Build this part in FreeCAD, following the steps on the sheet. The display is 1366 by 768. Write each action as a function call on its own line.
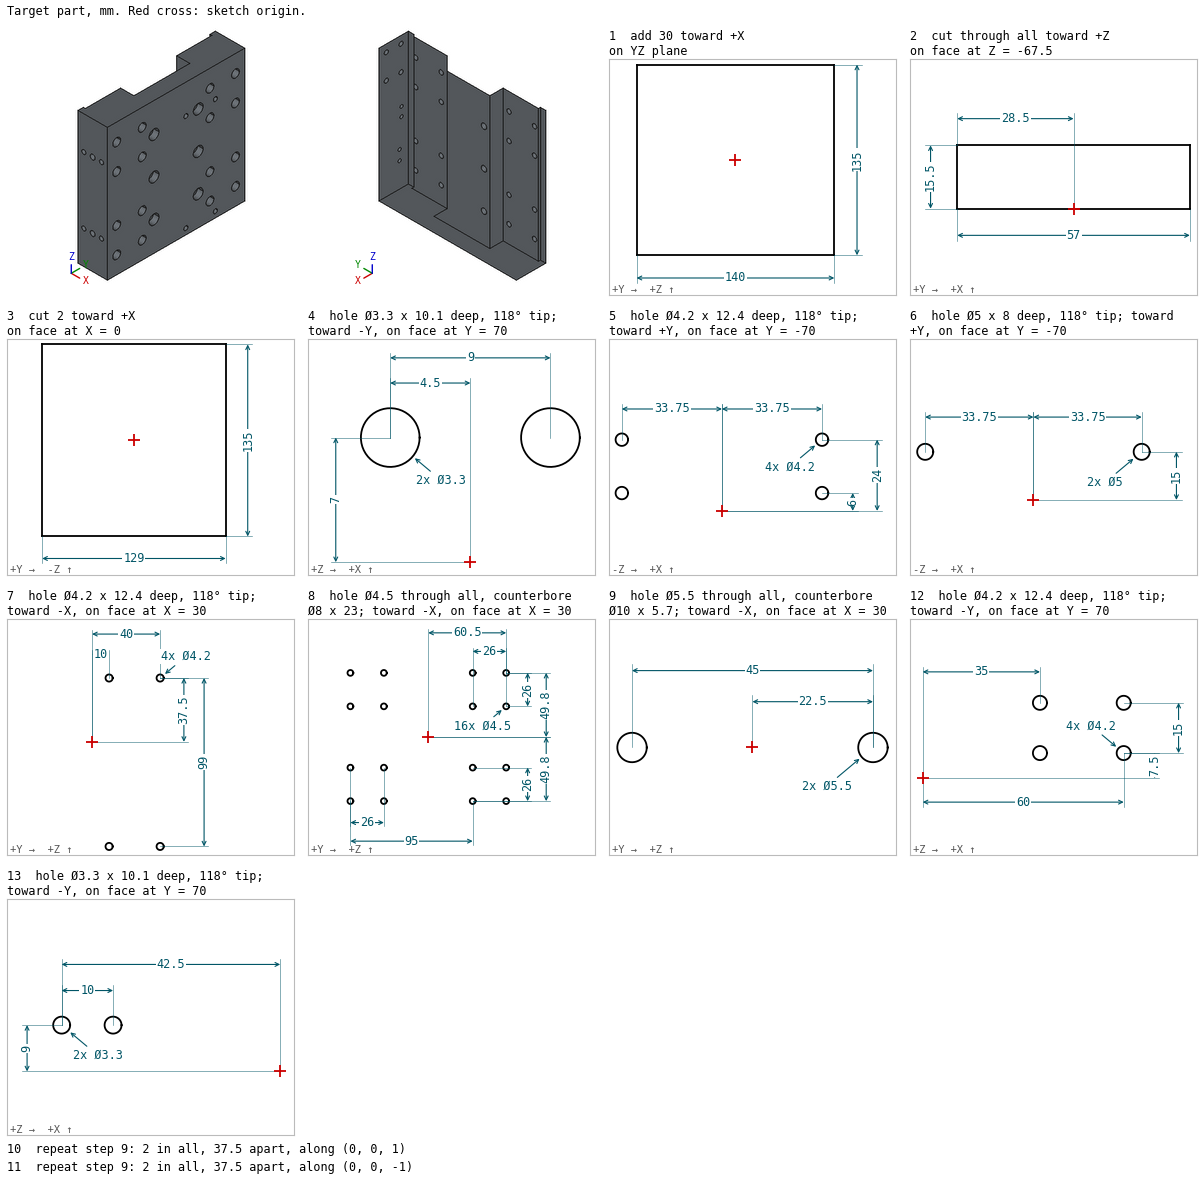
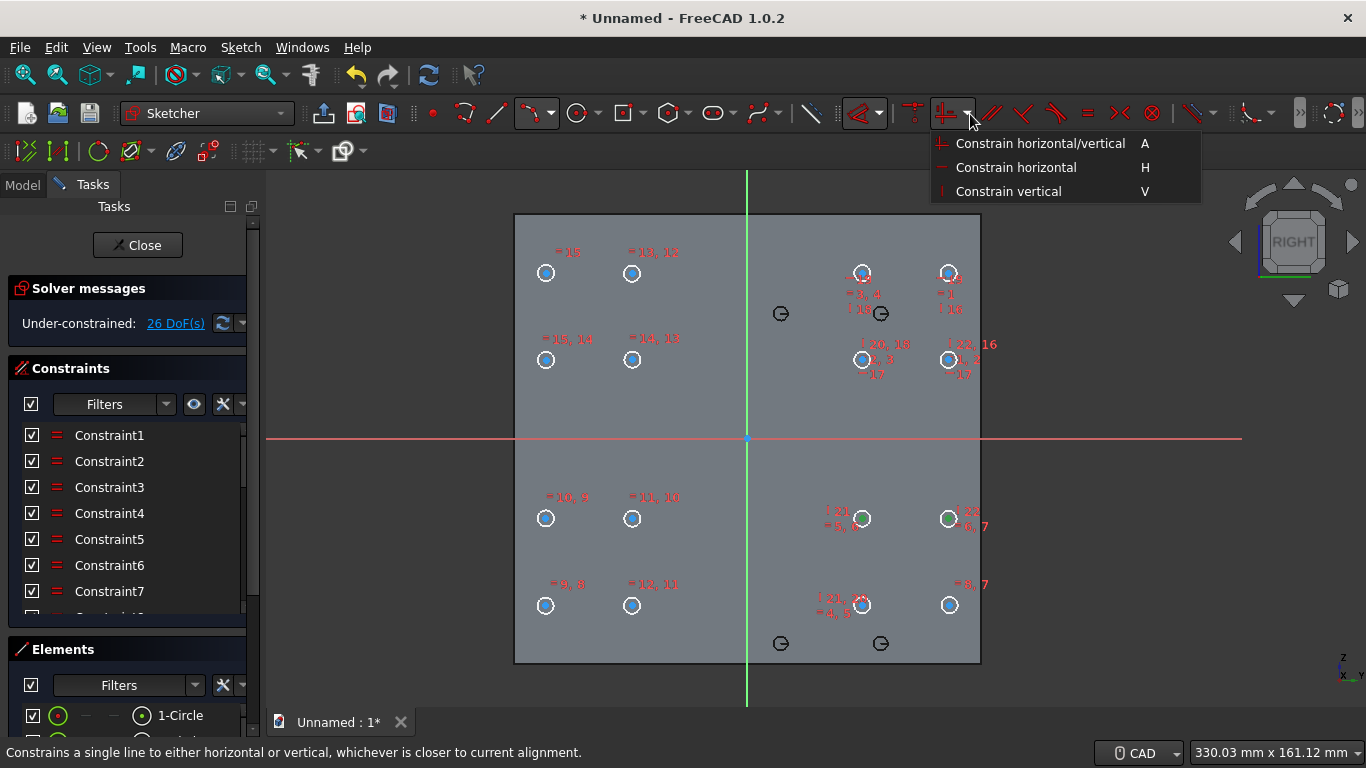
click(1066, 167)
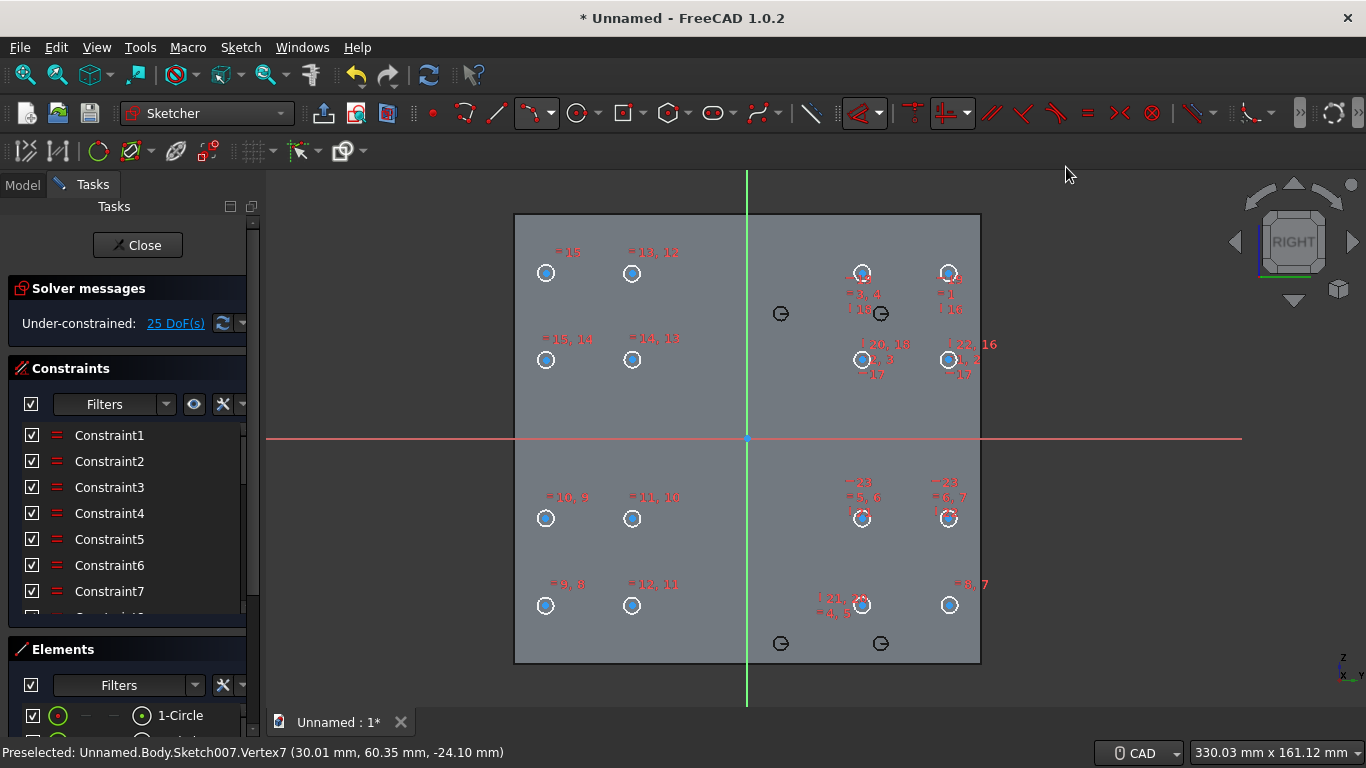
click(949, 519)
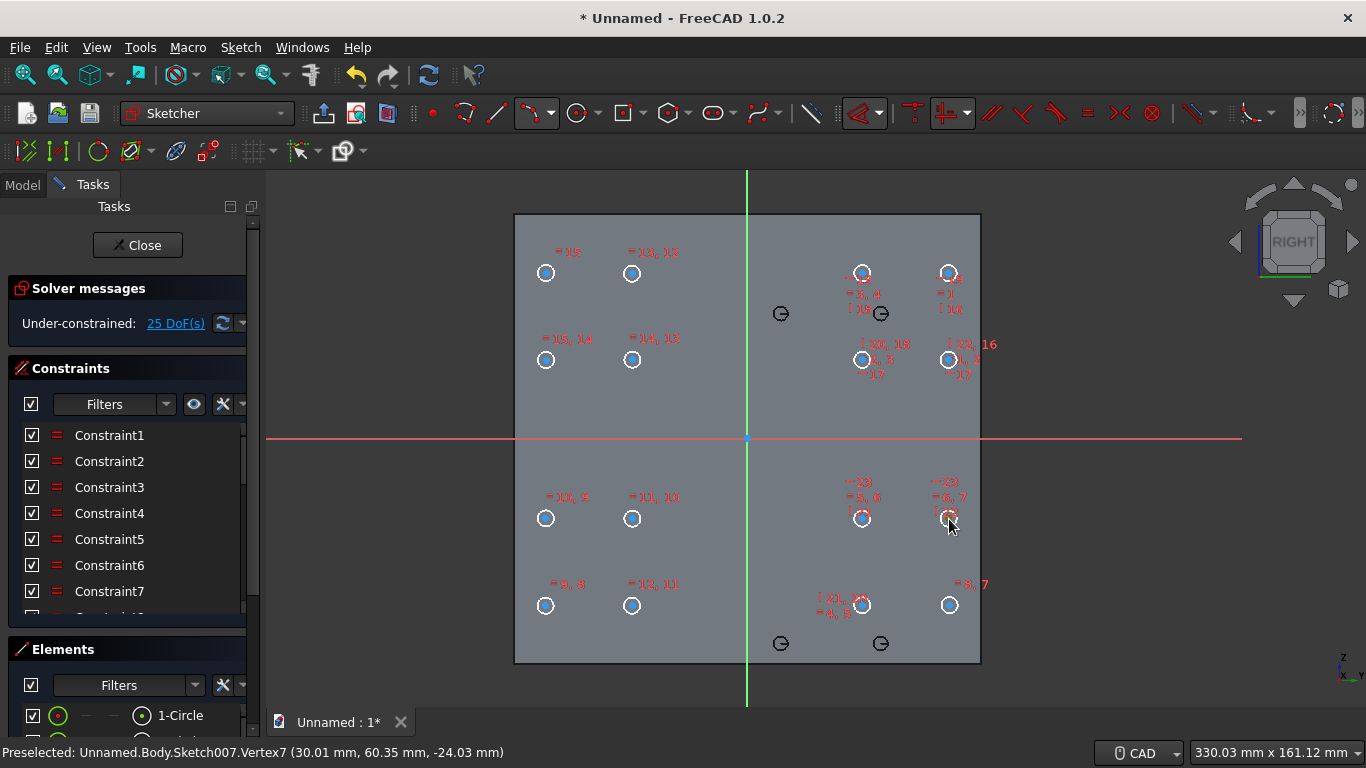
click(950, 605)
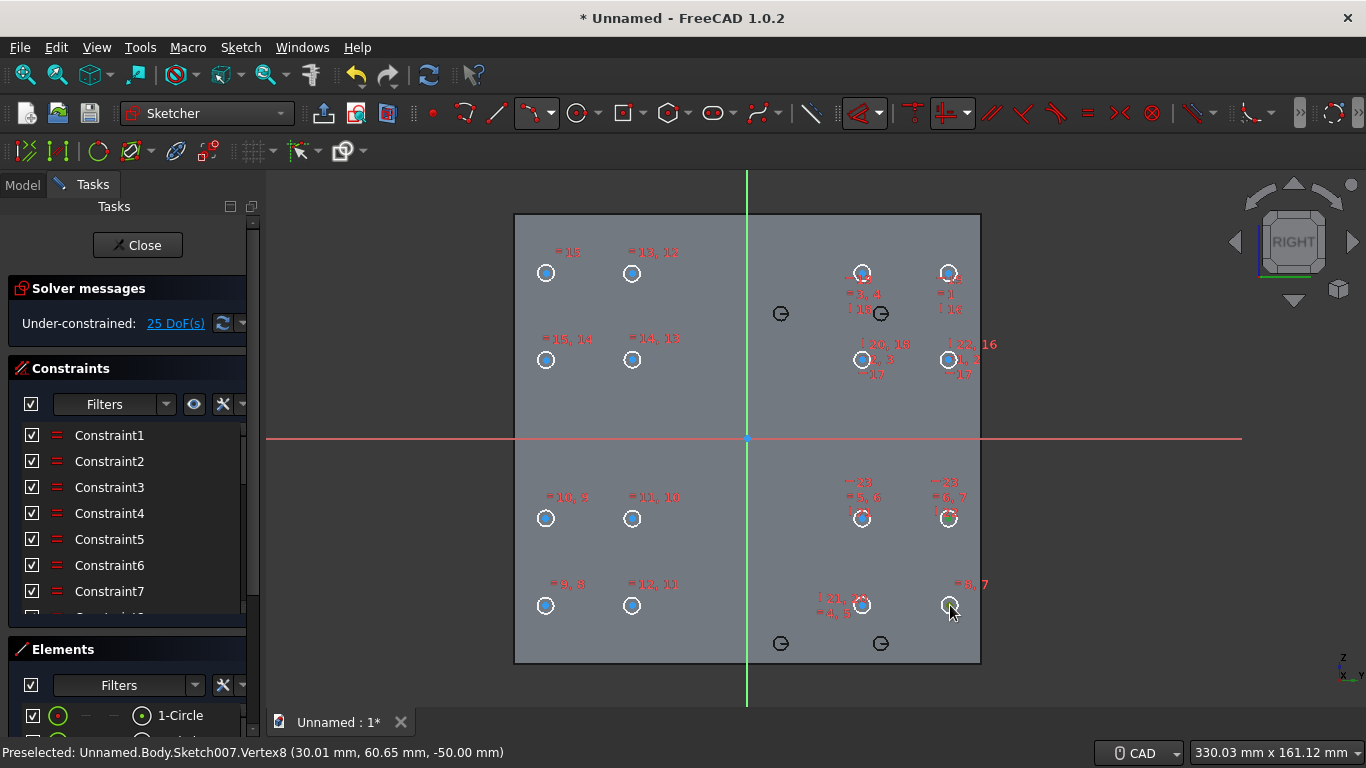
key(v)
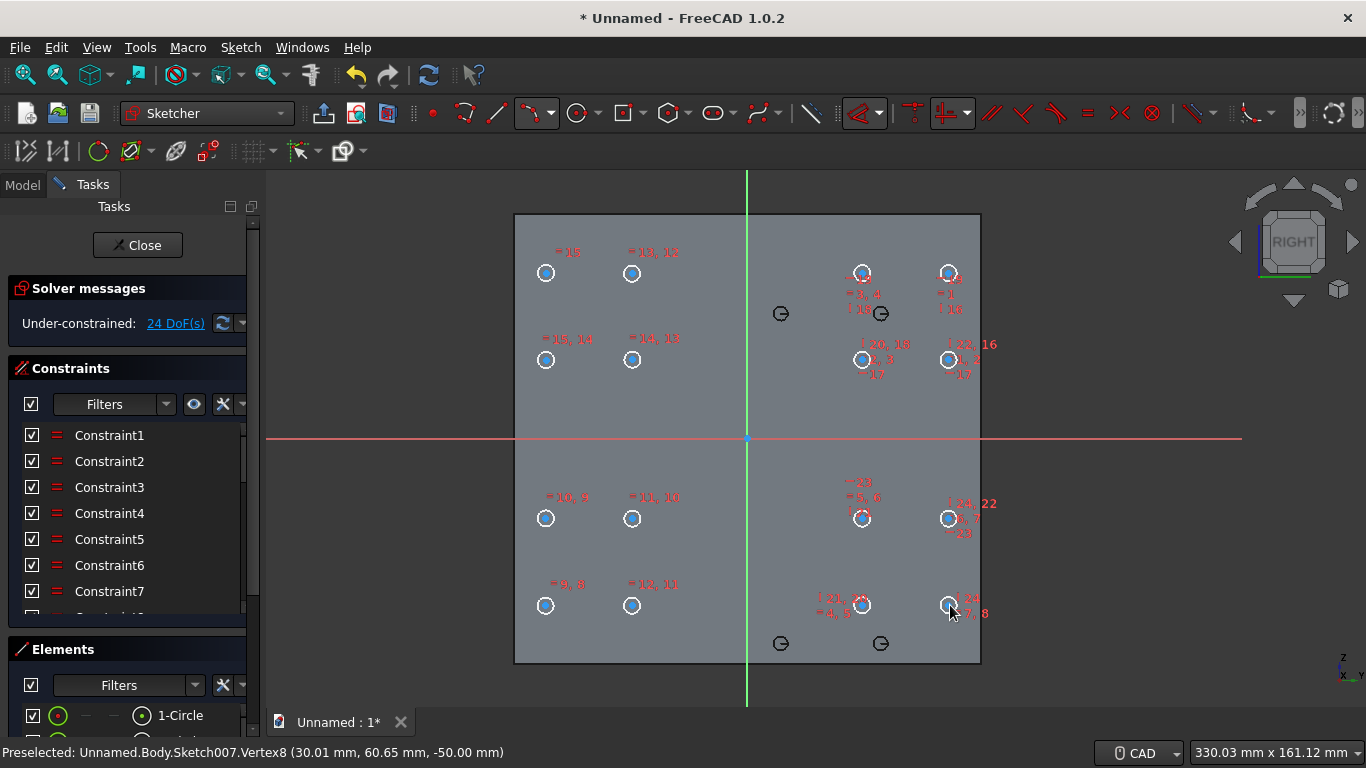
click(862, 605)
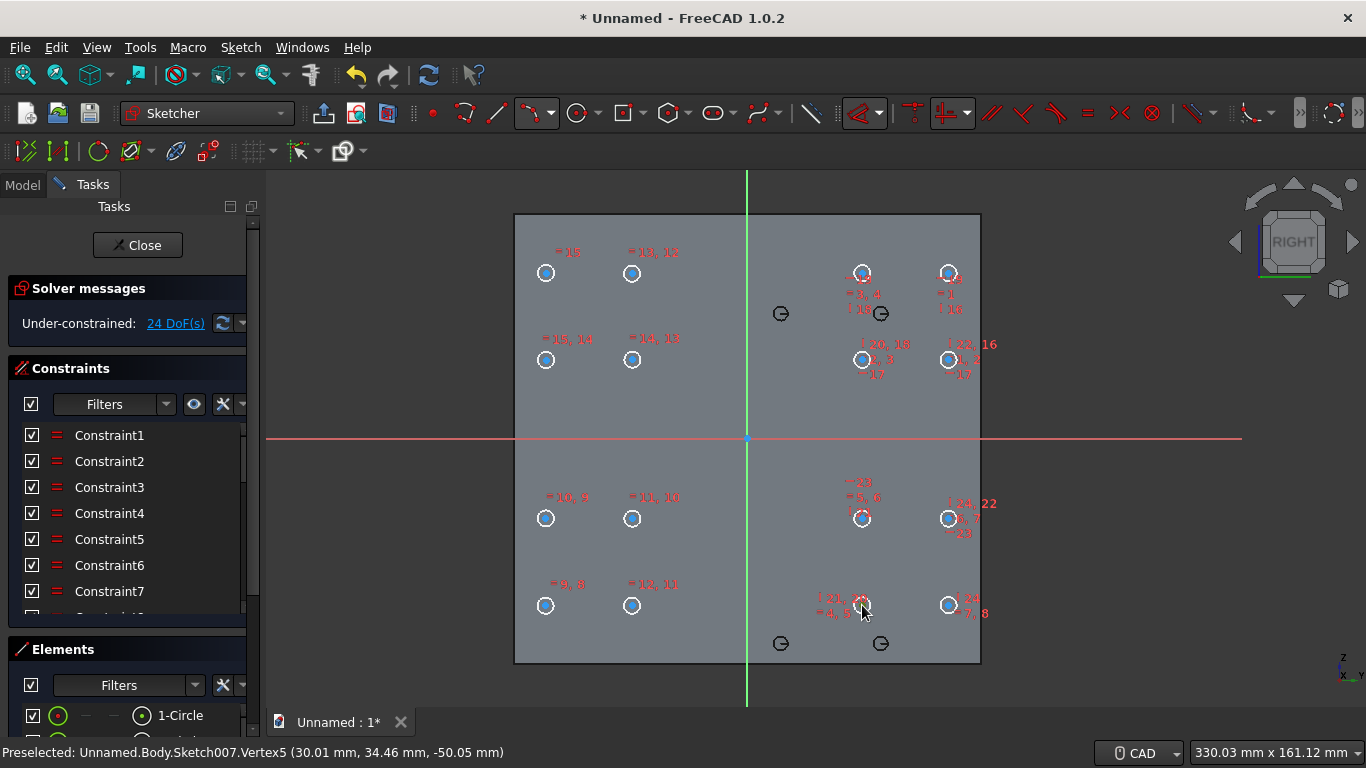
click(949, 605)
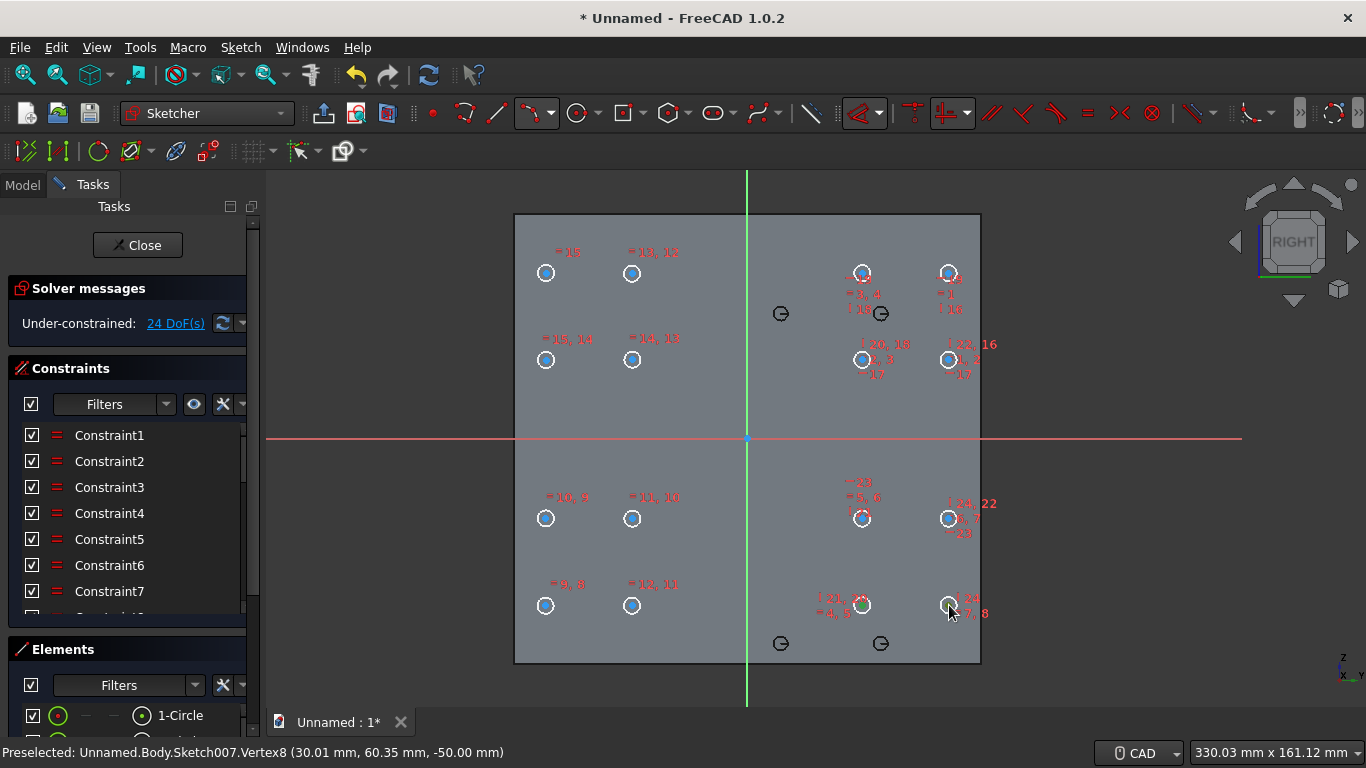
click(970, 114)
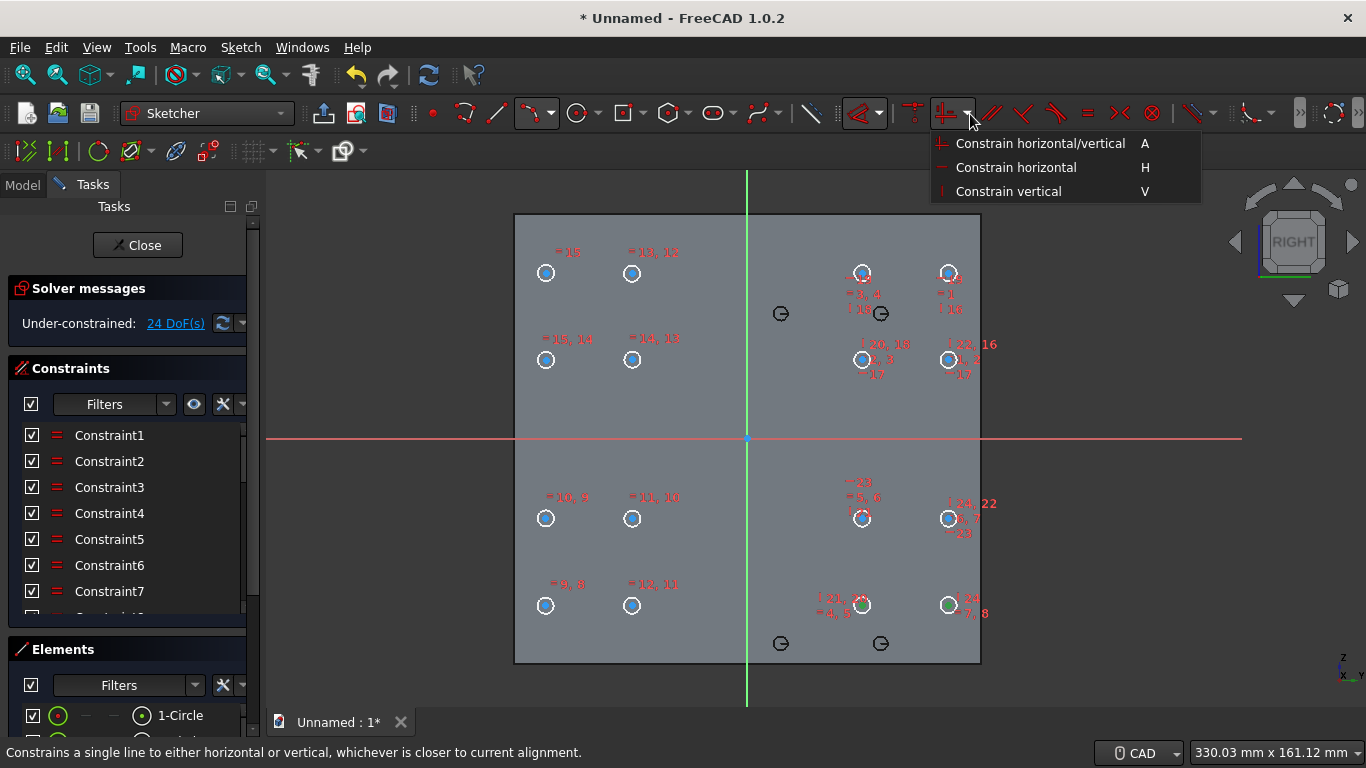
click(1066, 167)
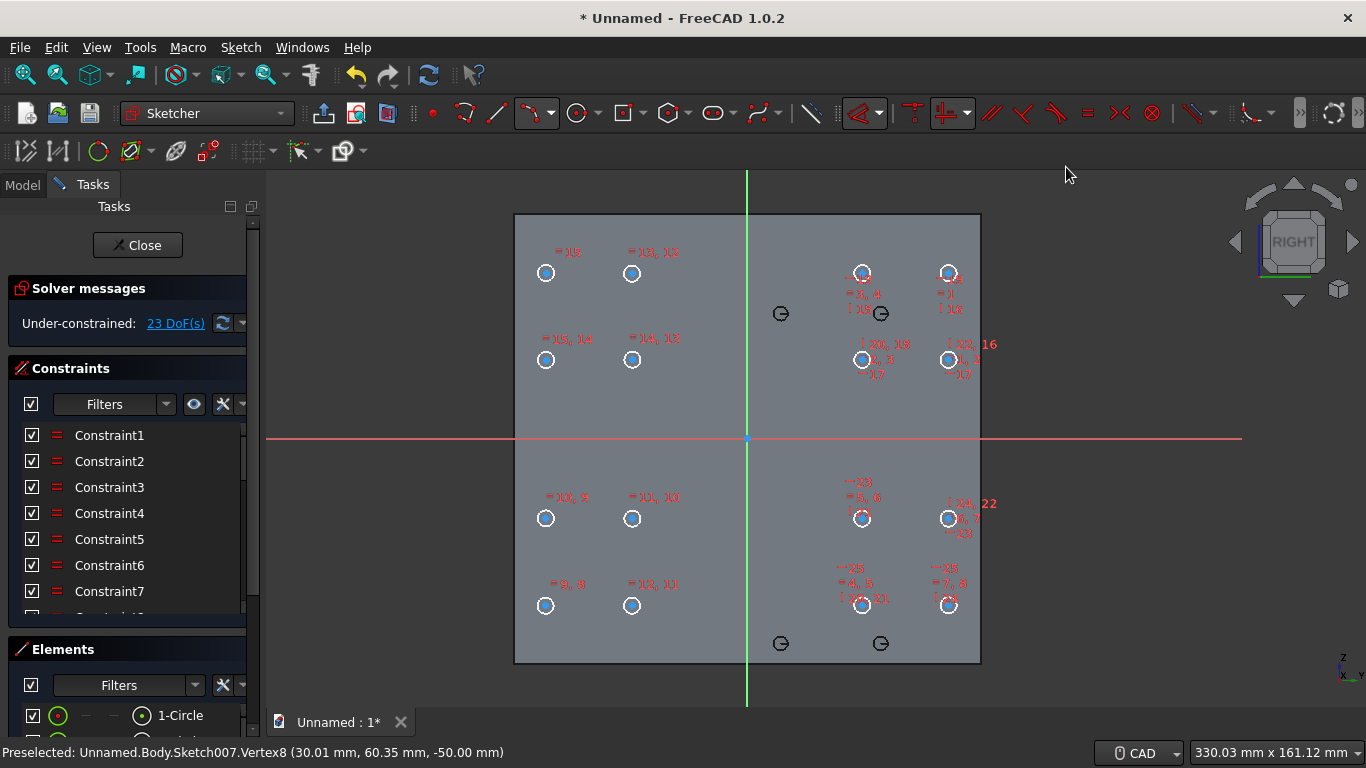
click(862, 605)